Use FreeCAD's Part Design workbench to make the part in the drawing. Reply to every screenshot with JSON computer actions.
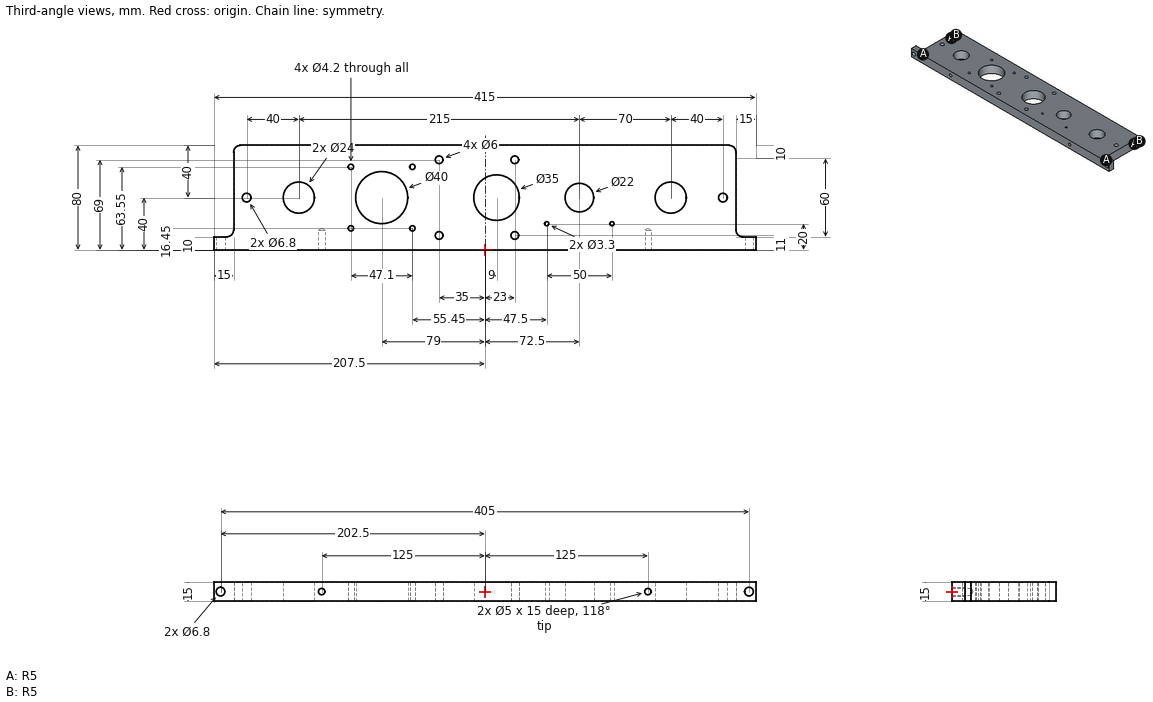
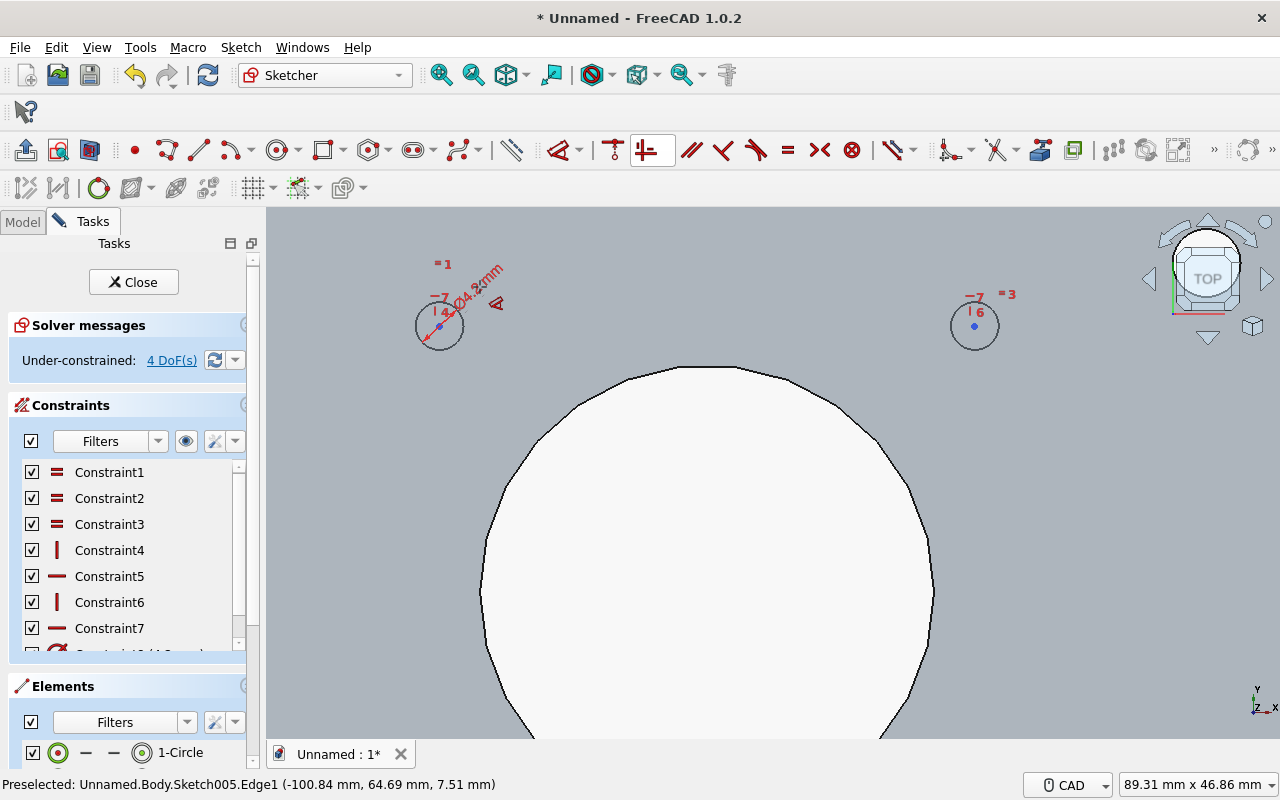
{"action": "left_click", "coordinate": [440, 326]}
{"action": "left_click", "coordinate": [406, 519]}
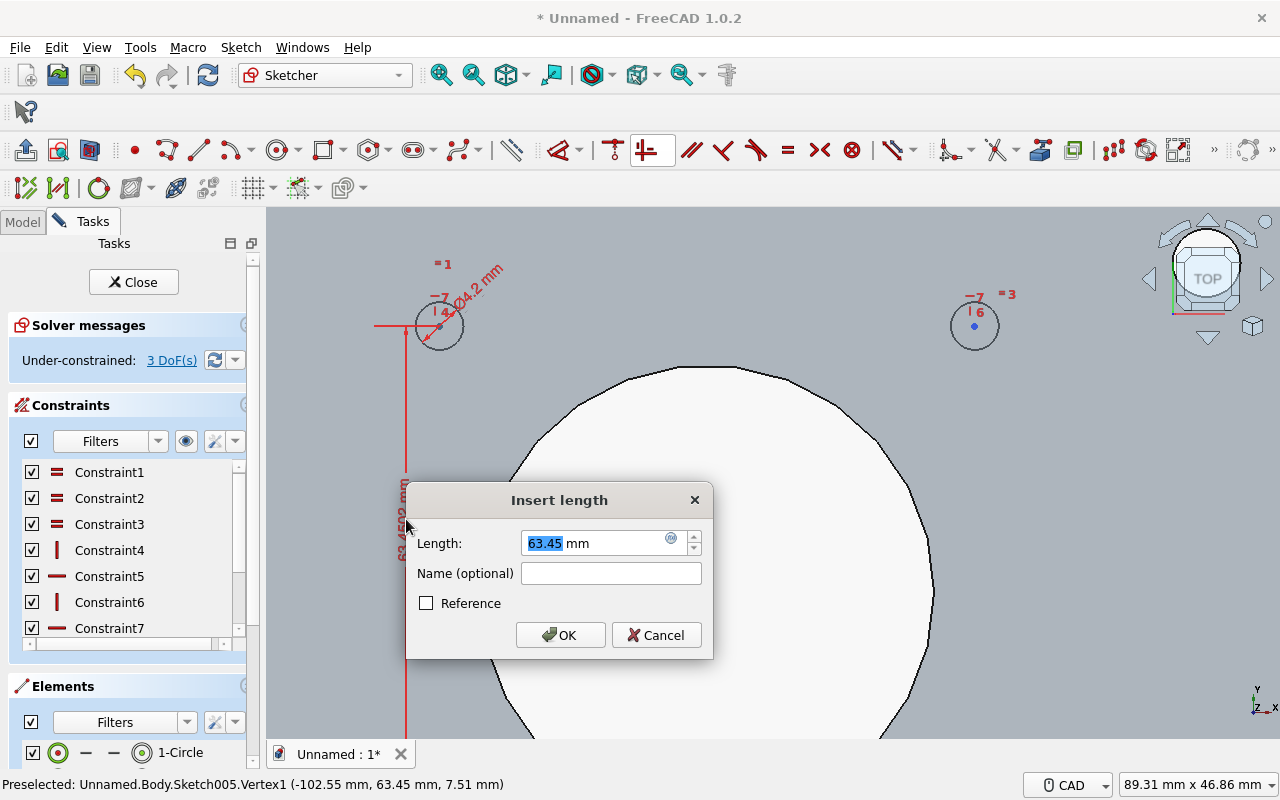
{"action": "type", "text": "63.55"}
{"action": "key", "text": "Return"}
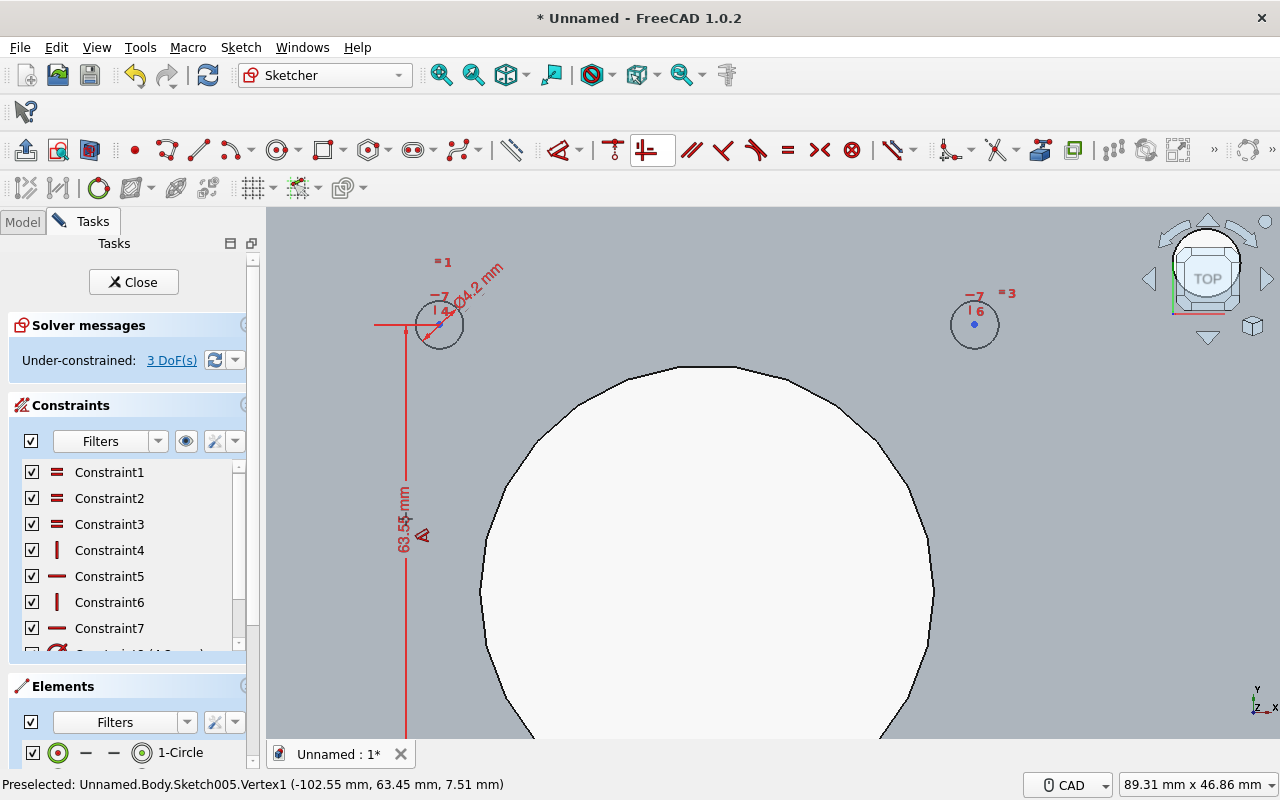
{"action": "scroll", "coordinate": [455, 309], "scroll_direction": "down", "scroll_amount": 4}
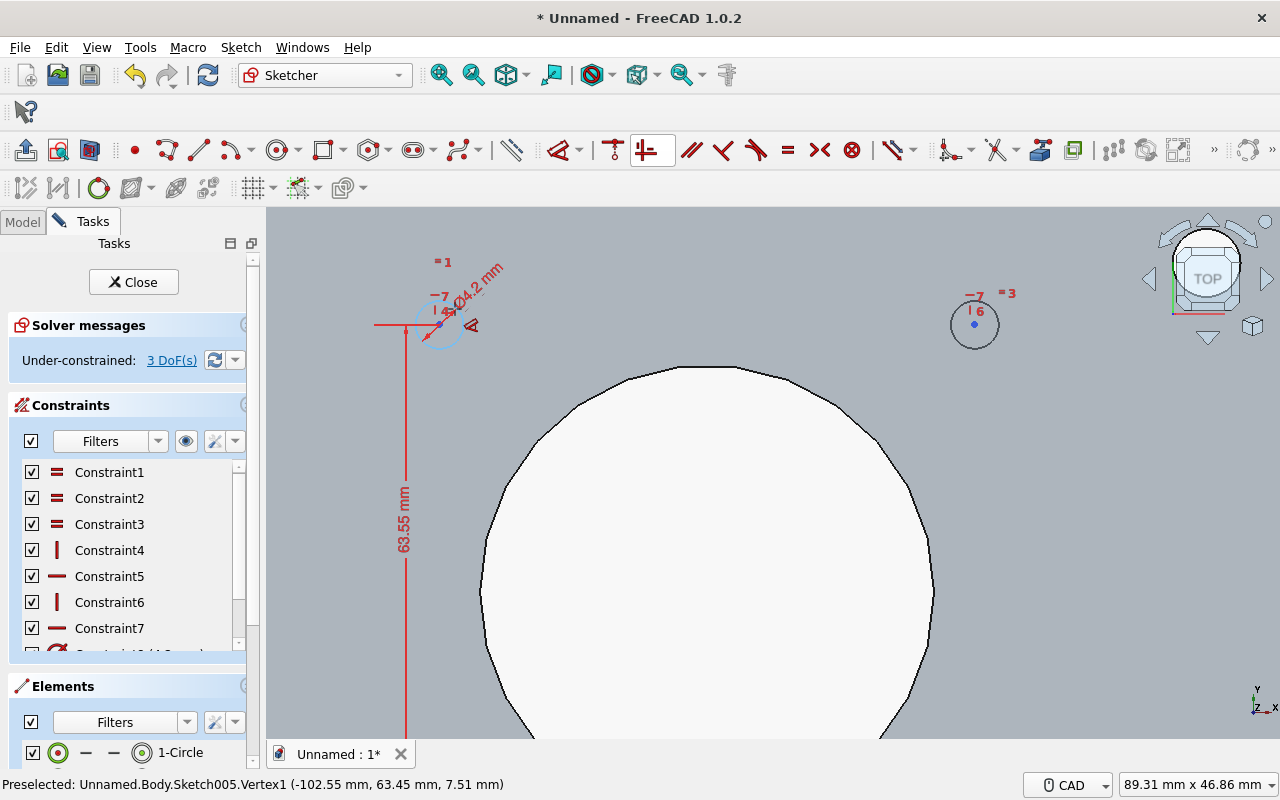
{"action": "left_click", "coordinate": [689, 557]}
{"action": "left_click", "coordinate": [830, 674]}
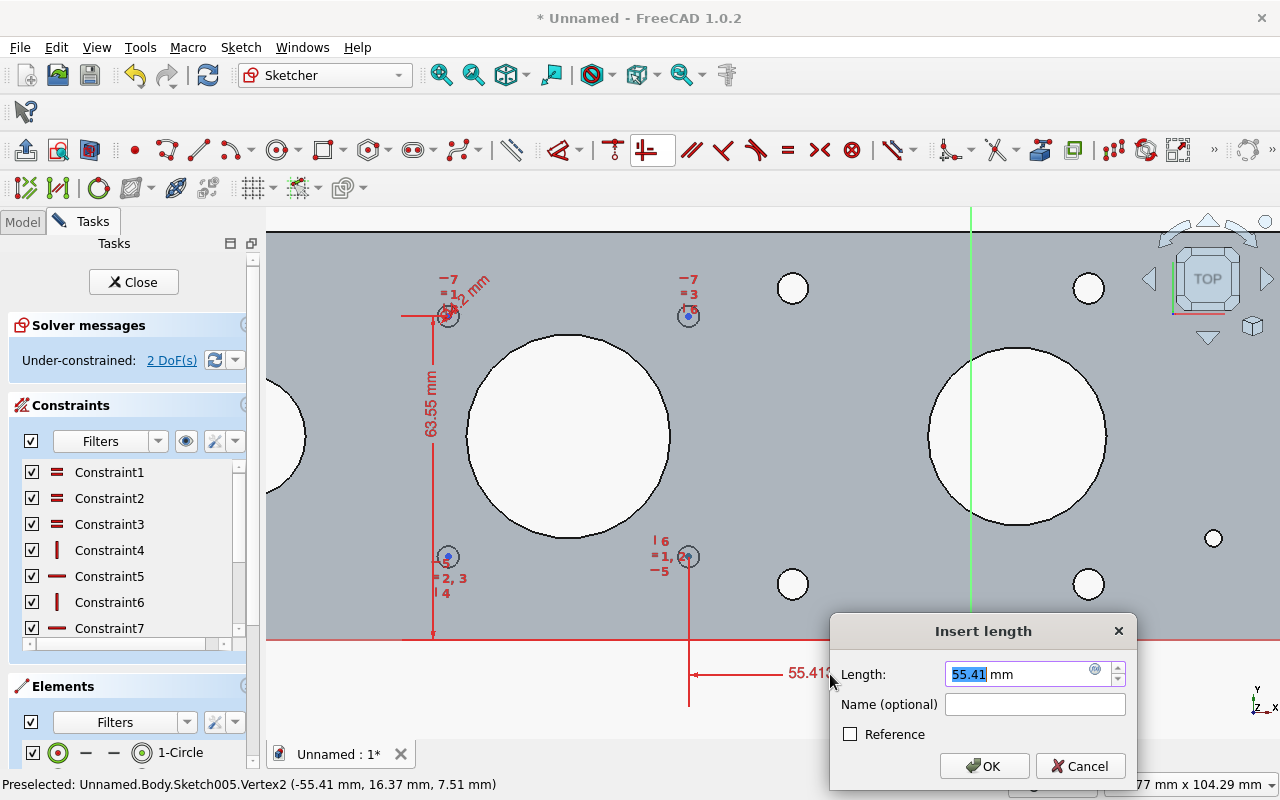
{"action": "type", "text": "55.45"}
{"action": "key", "text": "Return"}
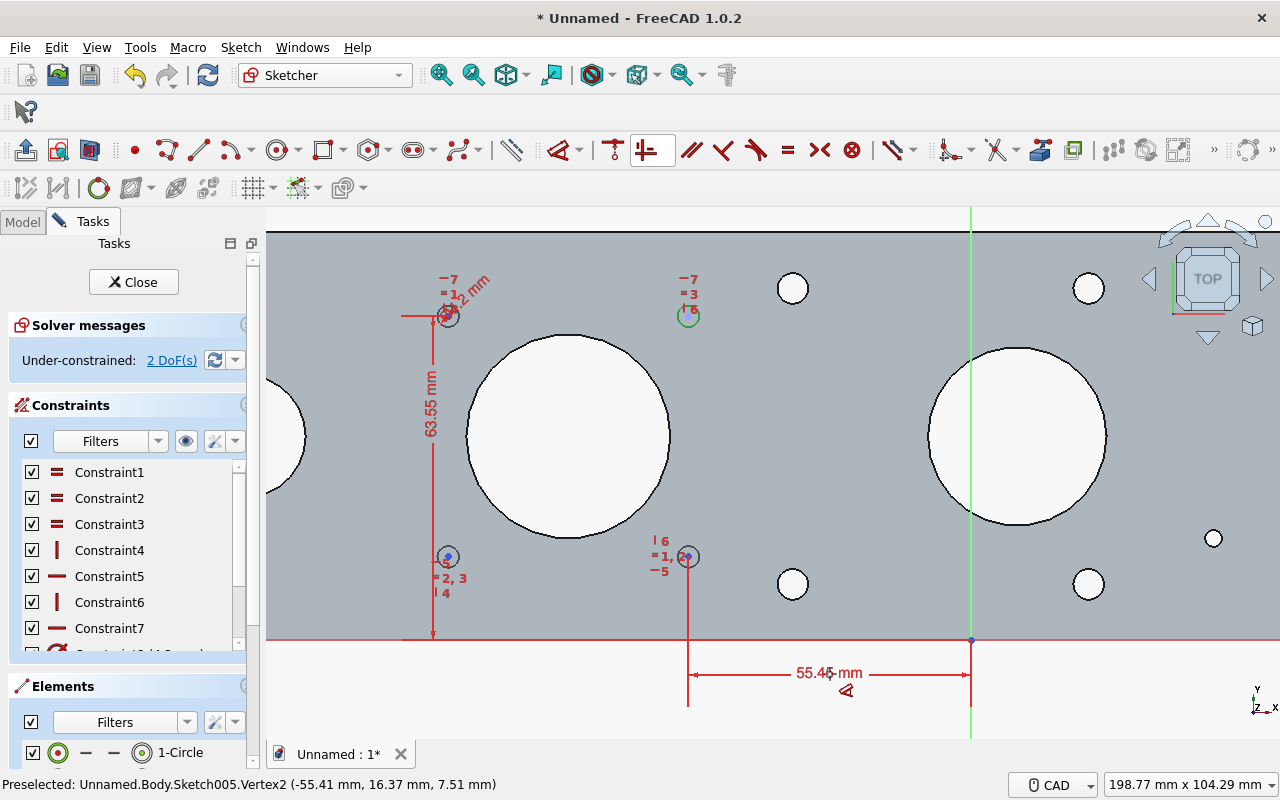
{"action": "left_click", "coordinate": [688, 557]}
{"action": "left_click", "coordinate": [1005, 599]}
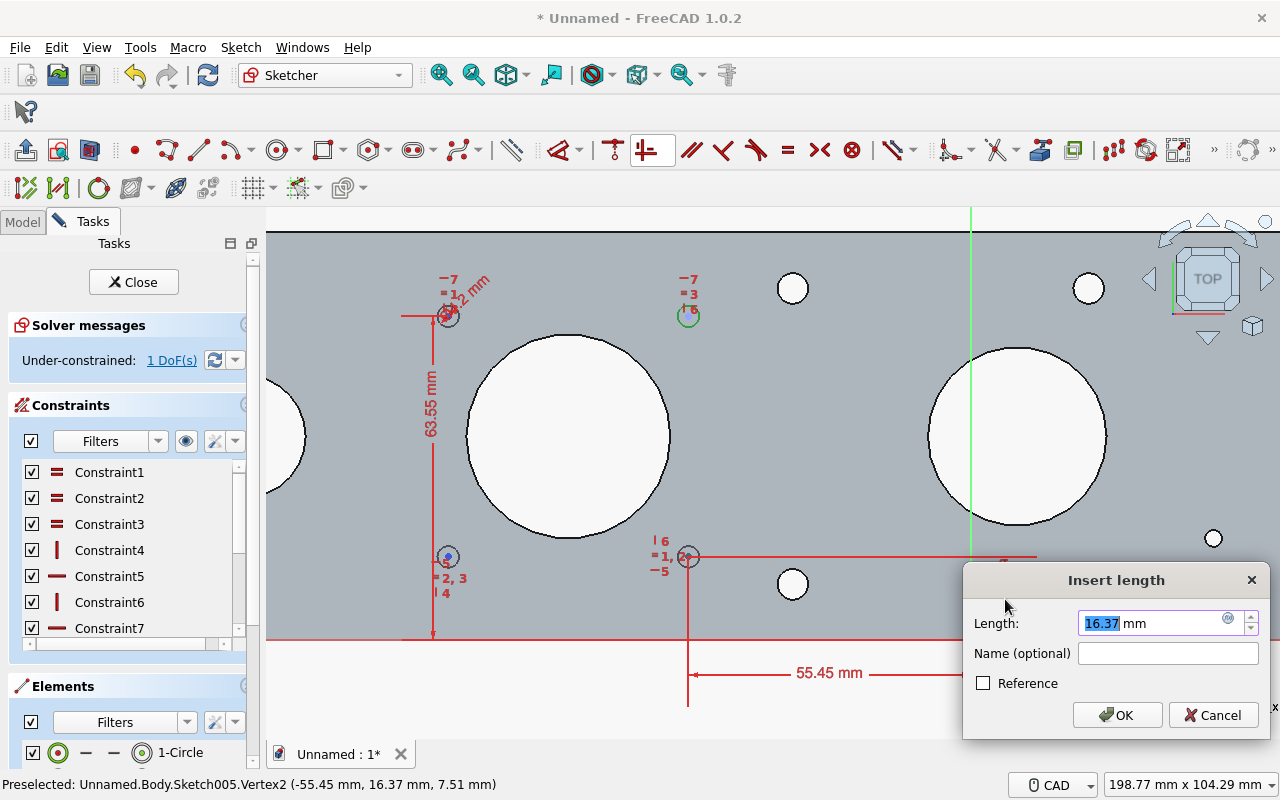
{"action": "type", "text": "16.45"}
{"action": "key", "text": "Return"}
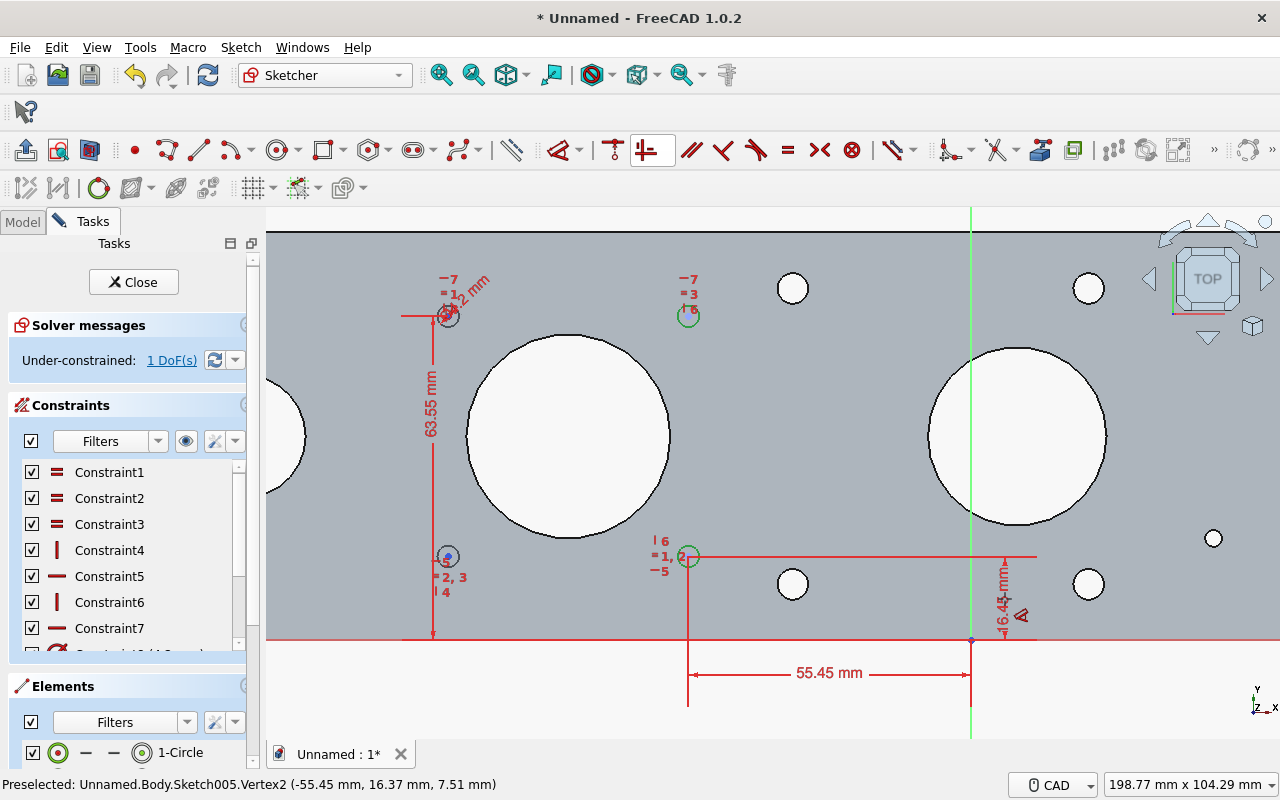
{"action": "left_click", "coordinate": [448, 316]}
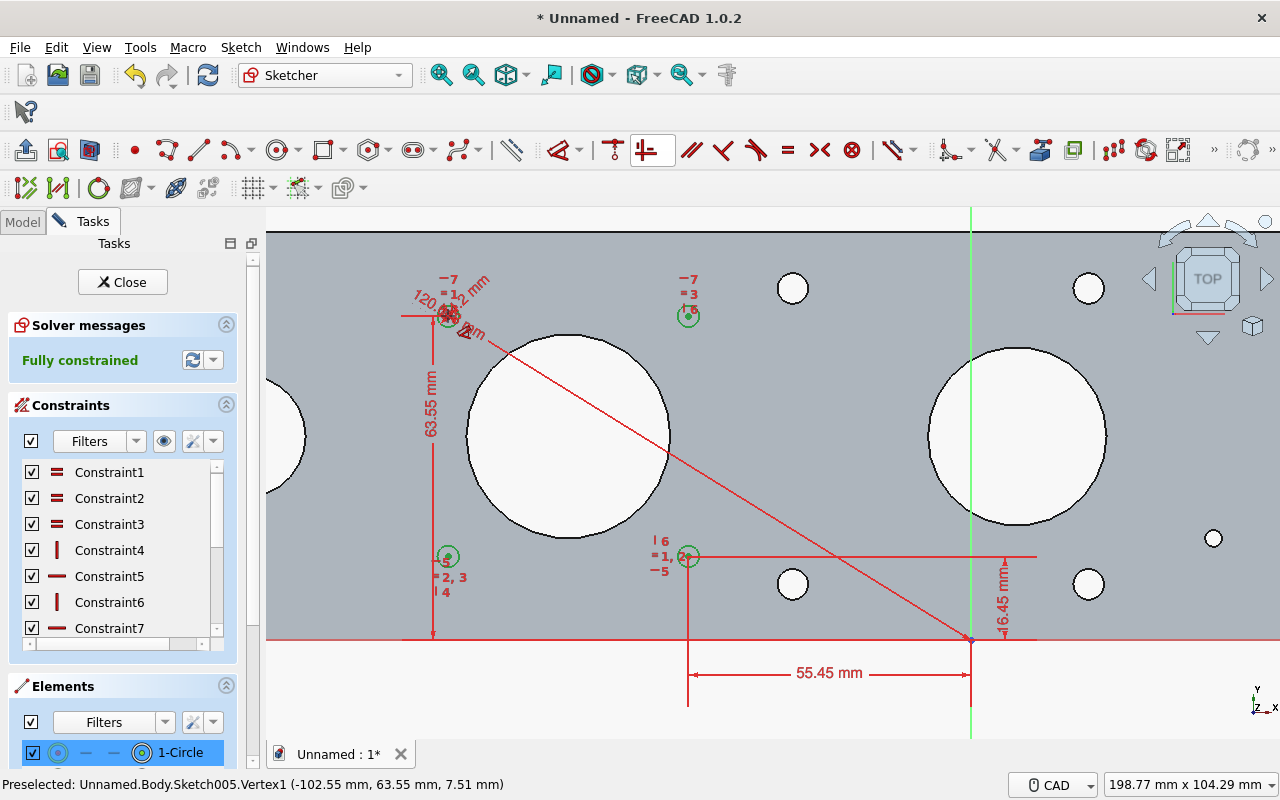
{"action": "left_click", "coordinate": [688, 557]}
{"action": "left_click", "coordinate": [568, 282]}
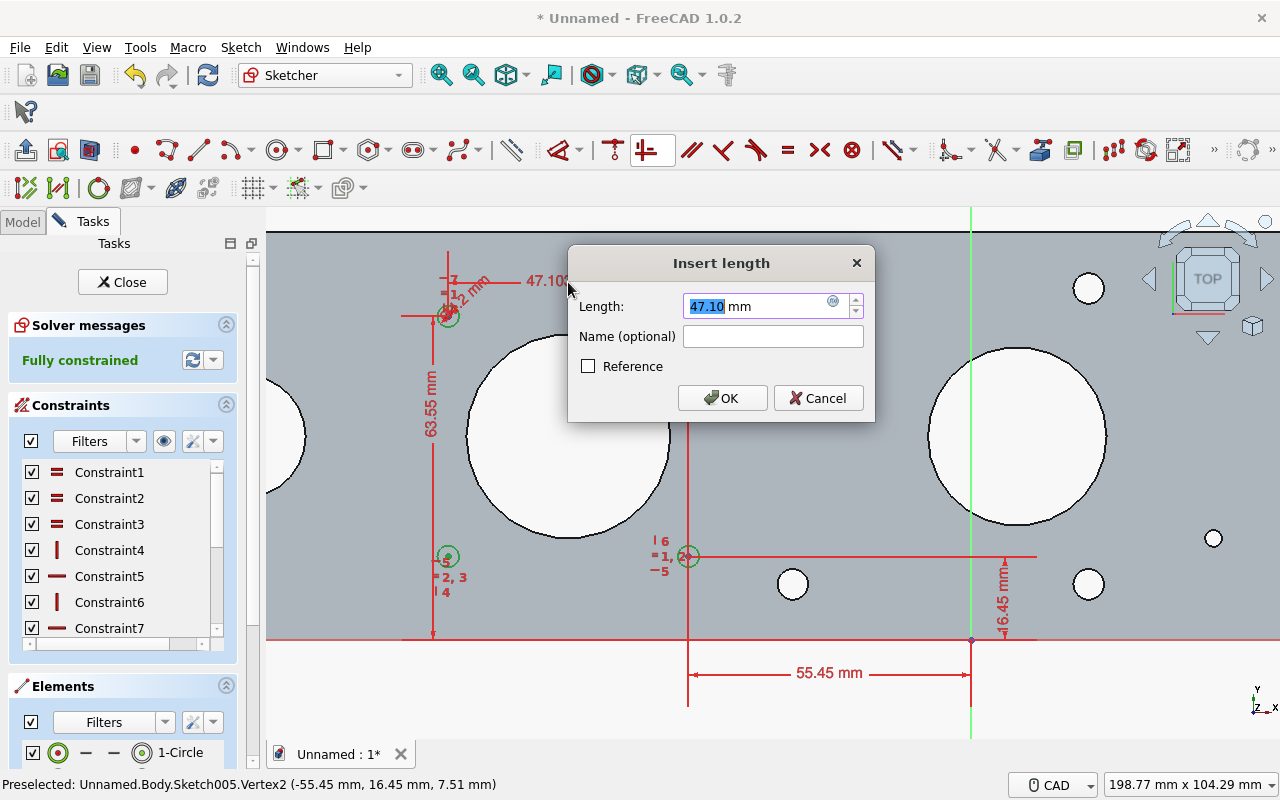
{"action": "type", "text": "47.1"}
{"action": "key", "text": "Return"}
{"action": "key", "text": "Escape"}